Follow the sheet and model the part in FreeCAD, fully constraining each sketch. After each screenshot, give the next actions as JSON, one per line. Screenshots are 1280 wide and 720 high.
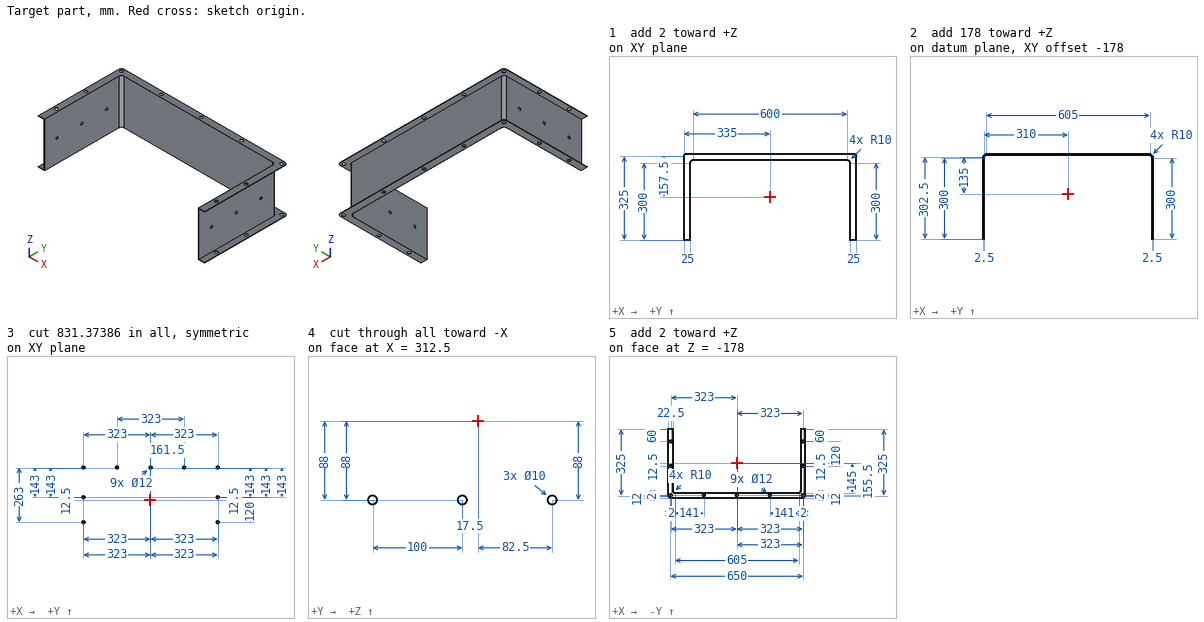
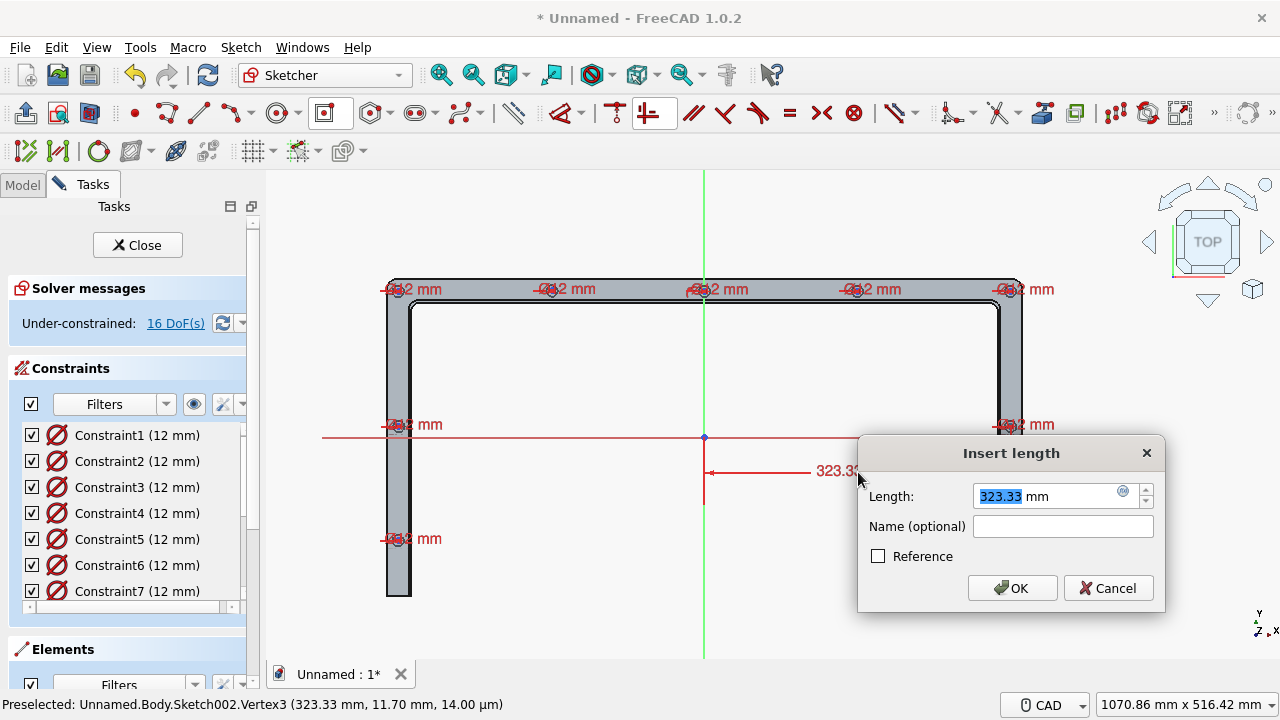
{"action": "type", "text": "323"}
{"action": "key", "text": "Return"}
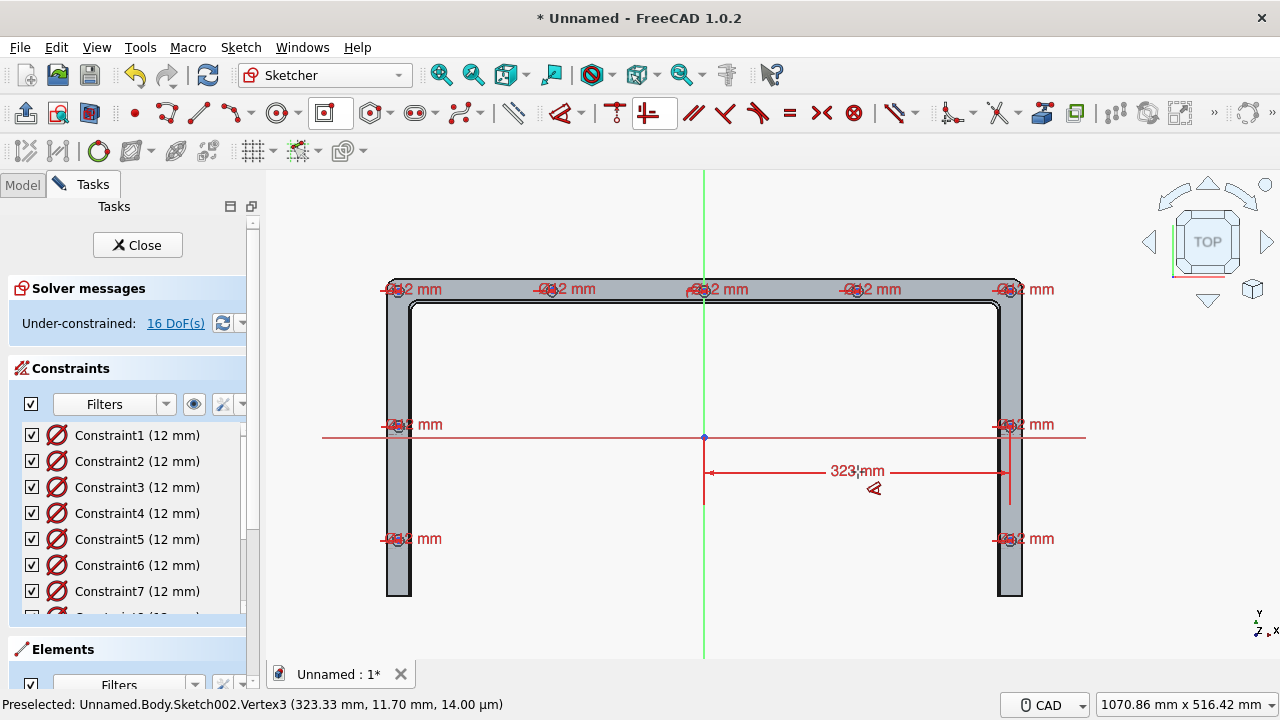
{"action": "left_click", "coordinate": [1010, 541]}
{"action": "left_click", "coordinate": [857, 575]}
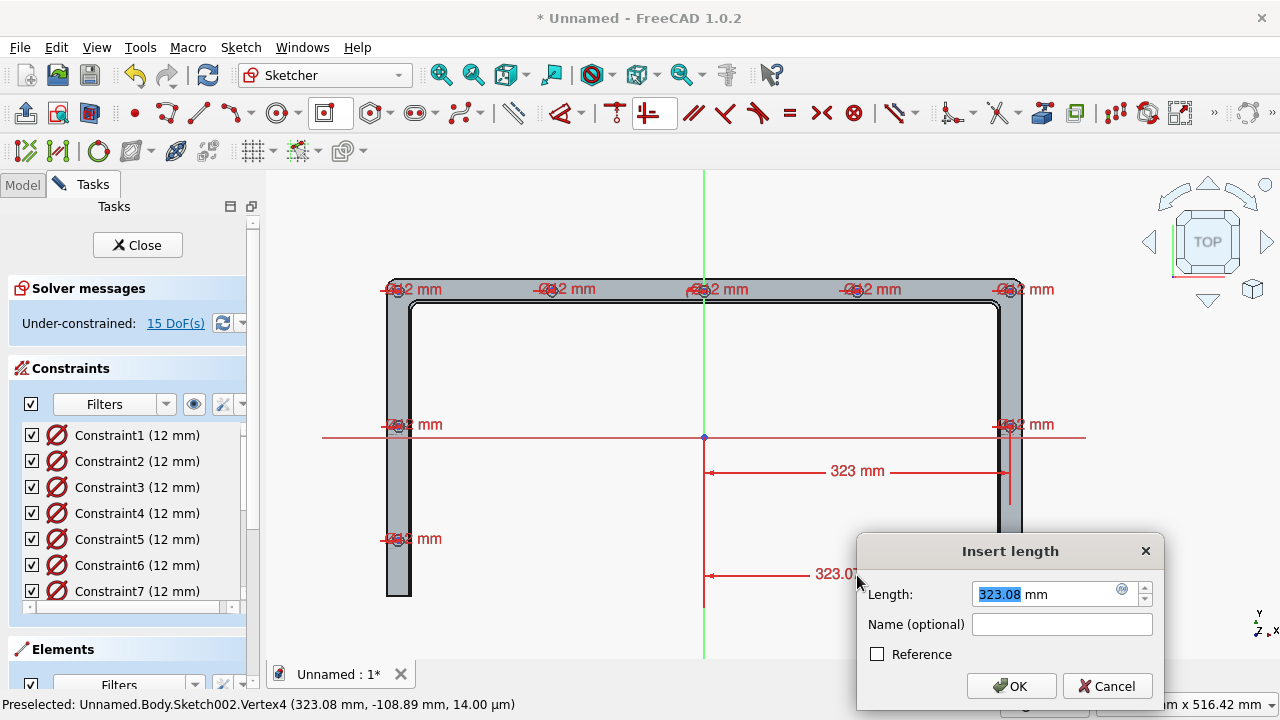
{"action": "type", "text": "323"}
{"action": "key", "text": "Return"}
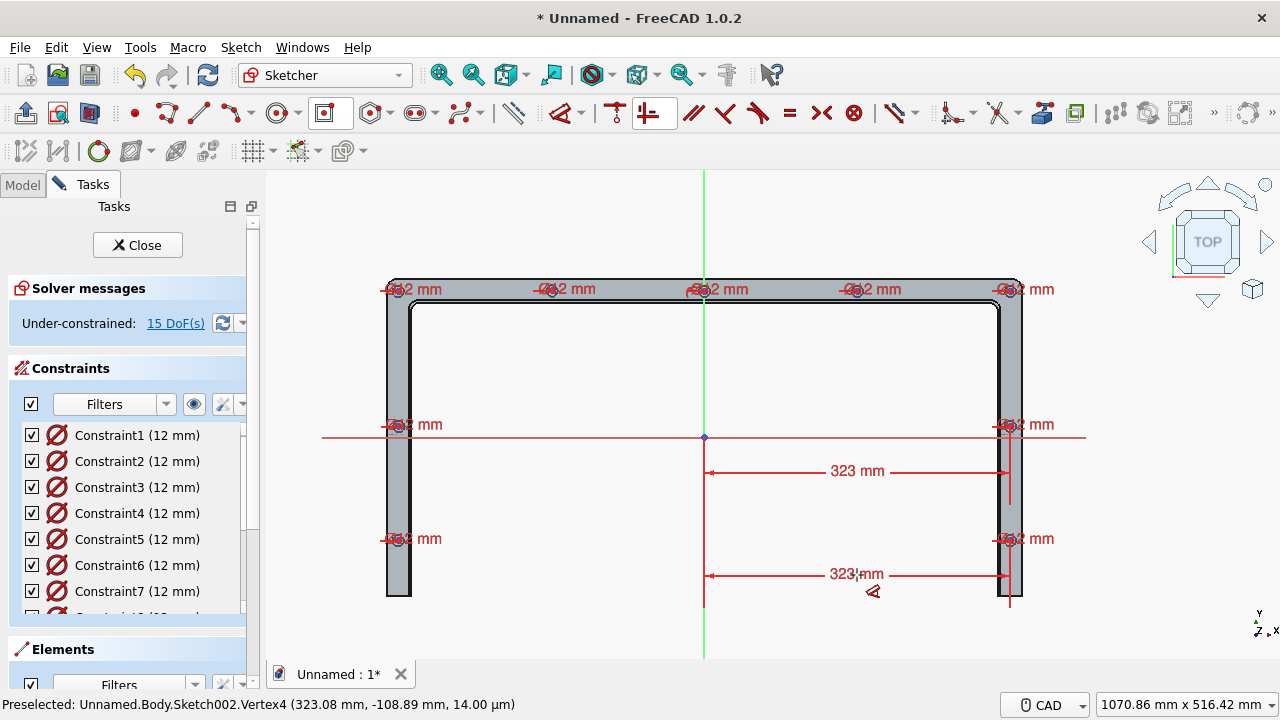
{"action": "left_click", "coordinate": [1010, 291]}
{"action": "left_click", "coordinate": [857, 257]}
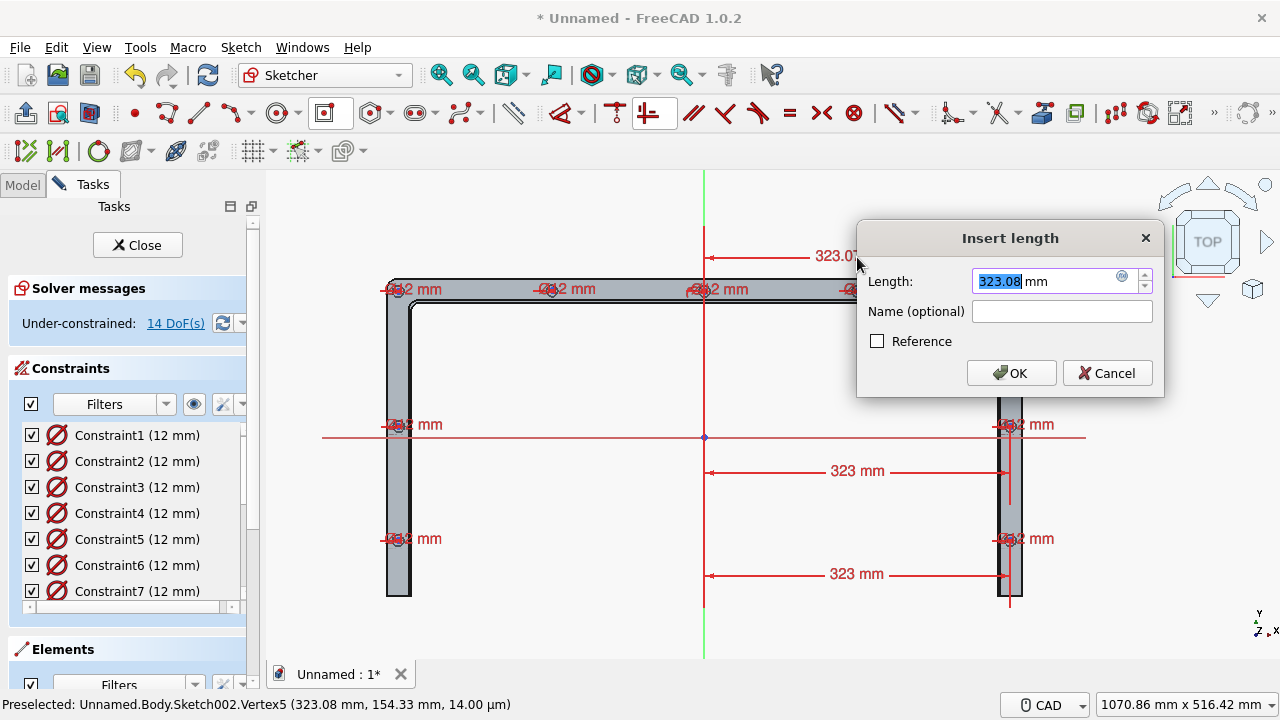
{"action": "type", "text": "323"}
{"action": "key", "text": "Return"}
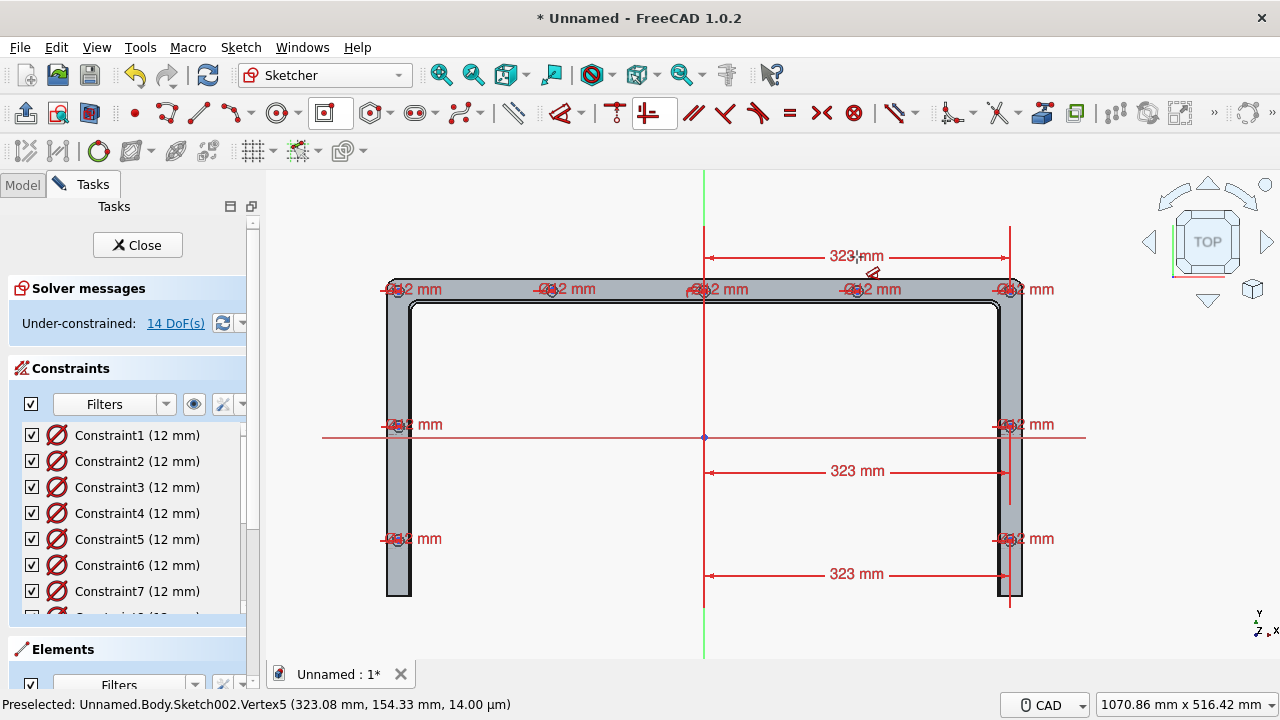
{"action": "left_click", "coordinate": [398, 291]}
{"action": "left_click", "coordinate": [551, 257]}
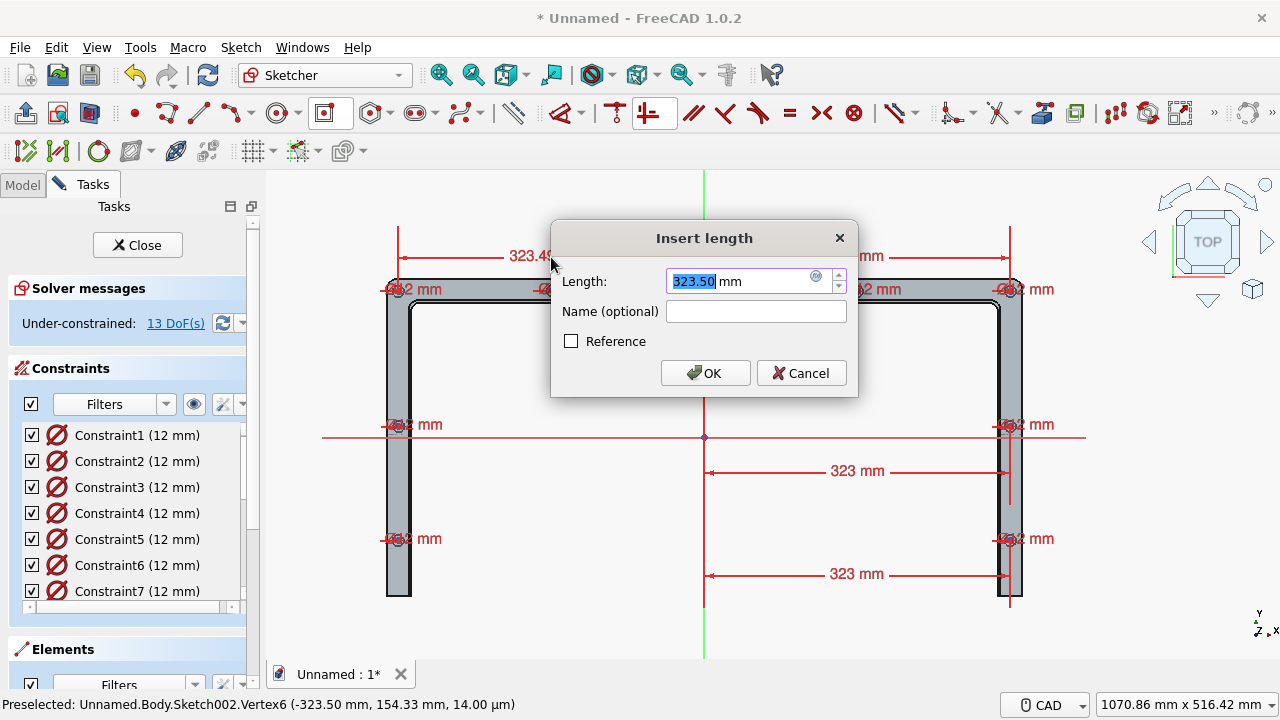
{"action": "type", "text": "323"}
{"action": "key", "text": "Return"}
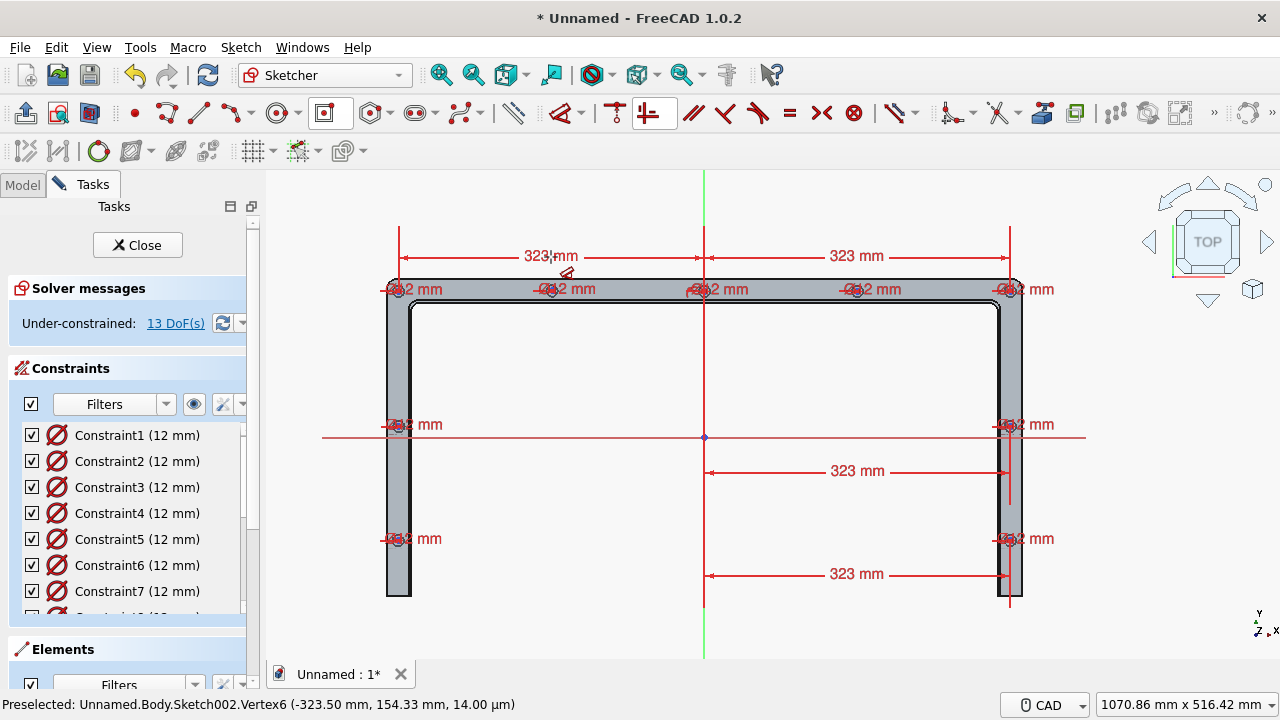
{"action": "left_click", "coordinate": [398, 541]}
{"action": "left_click", "coordinate": [551, 575]}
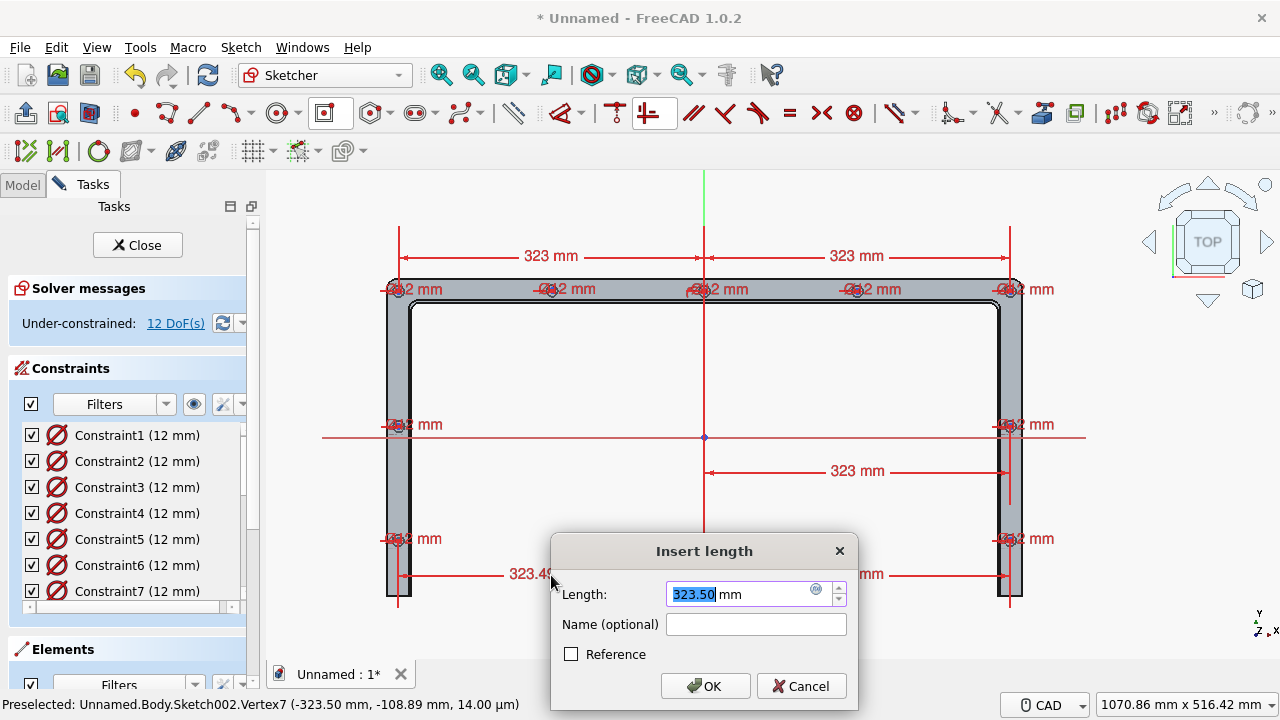
{"action": "type", "text": "323"}
{"action": "key", "text": "Return"}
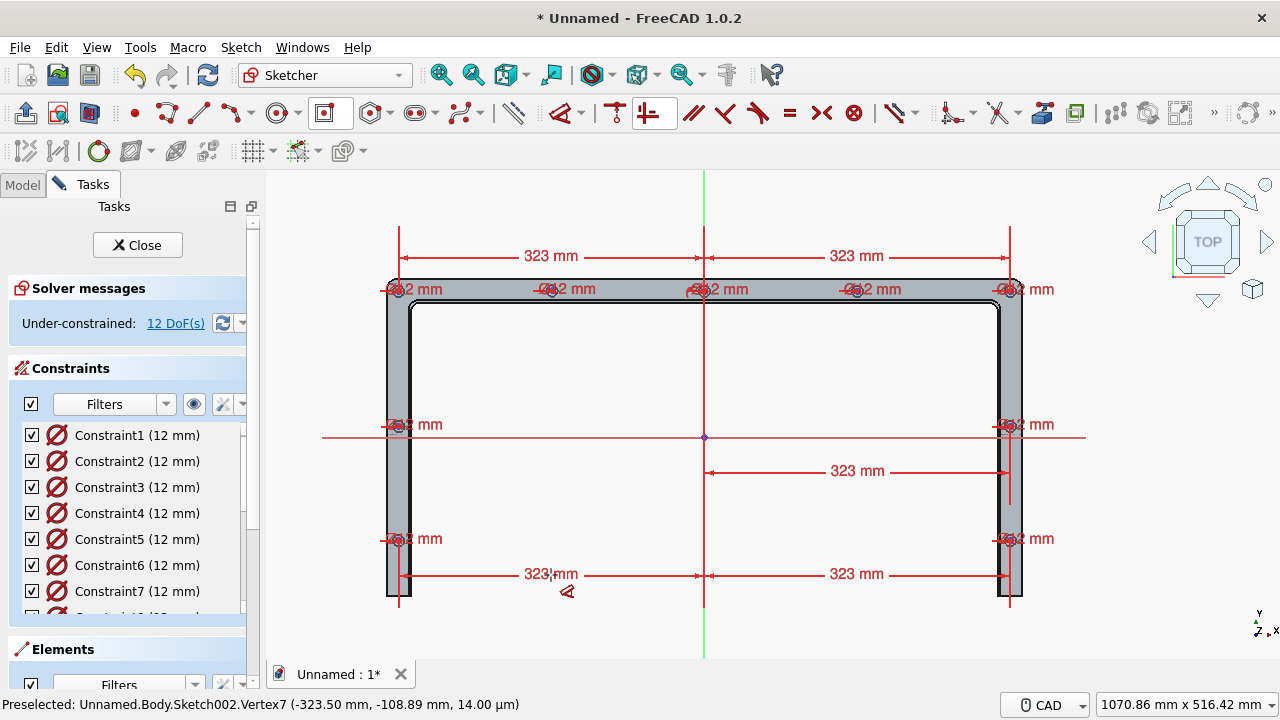
{"action": "left_click", "coordinate": [399, 427]}
{"action": "left_click", "coordinate": [552, 472]}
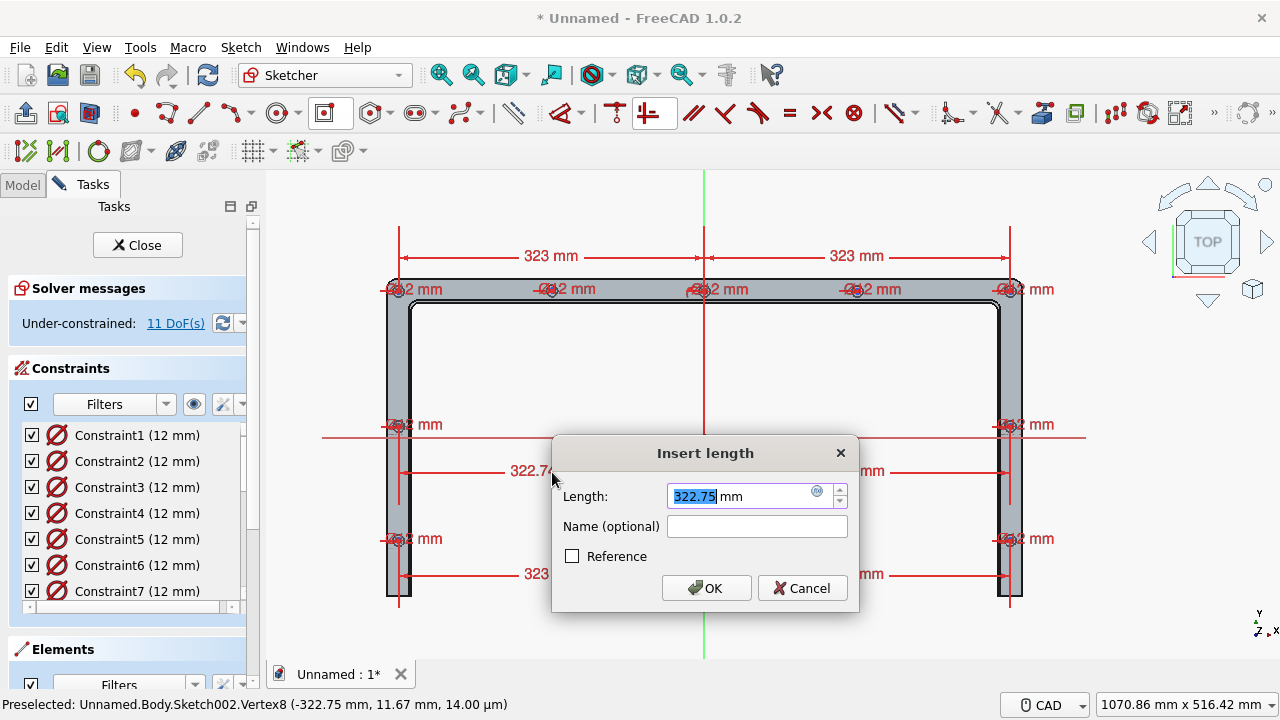
{"action": "type", "text": "323"}
{"action": "key", "text": "Return"}